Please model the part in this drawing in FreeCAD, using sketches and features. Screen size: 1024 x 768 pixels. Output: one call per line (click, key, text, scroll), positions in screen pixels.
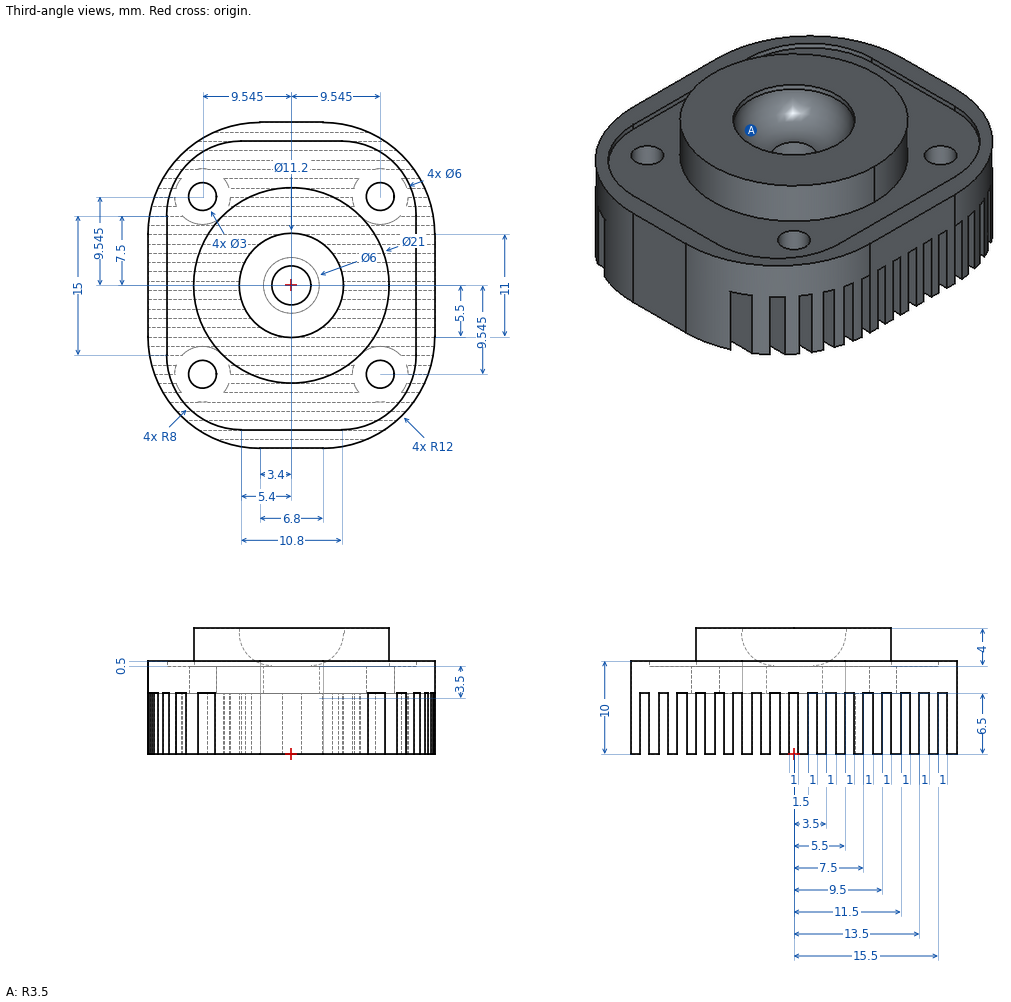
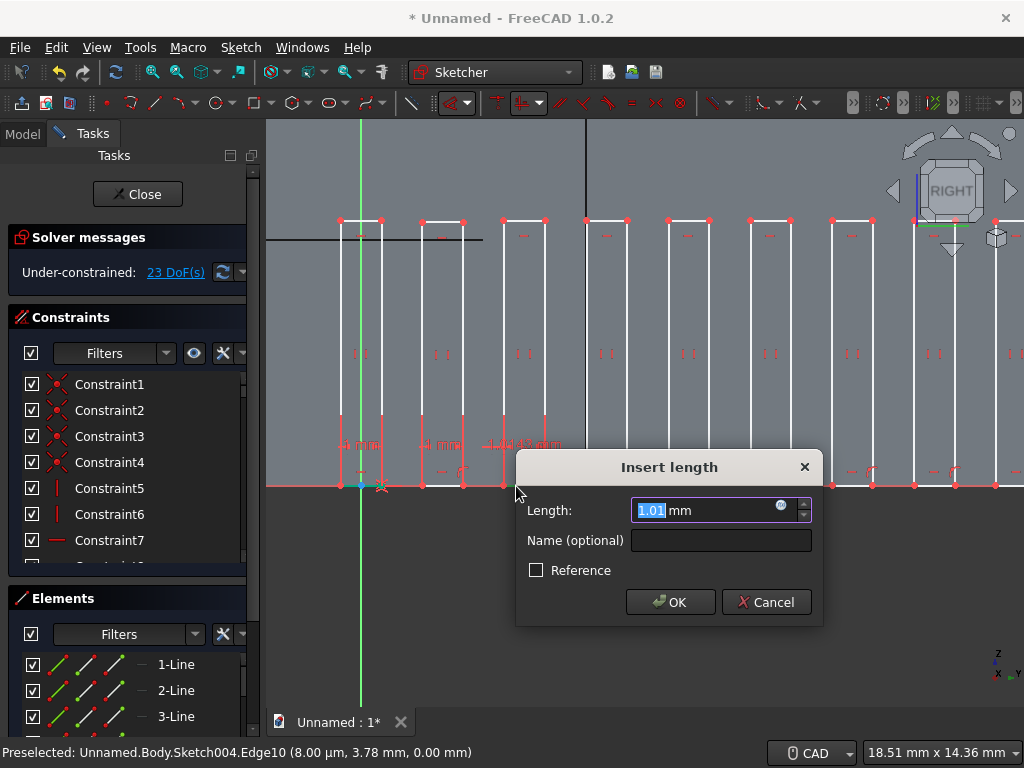
text(1)
key(Return)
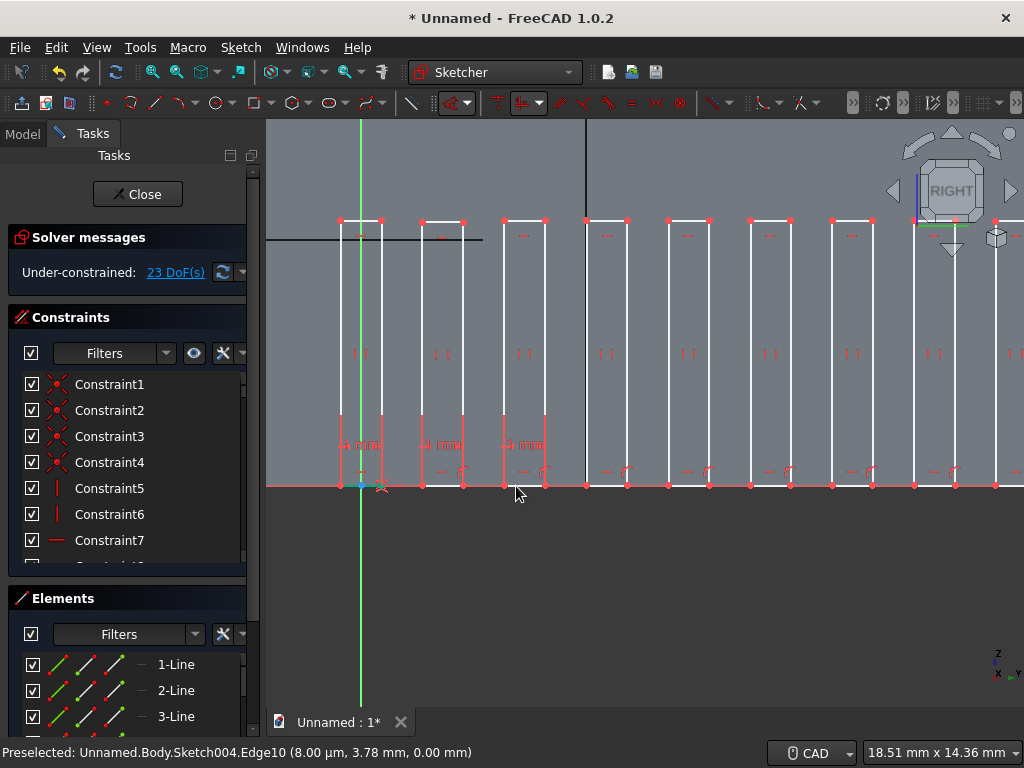
click(599, 486)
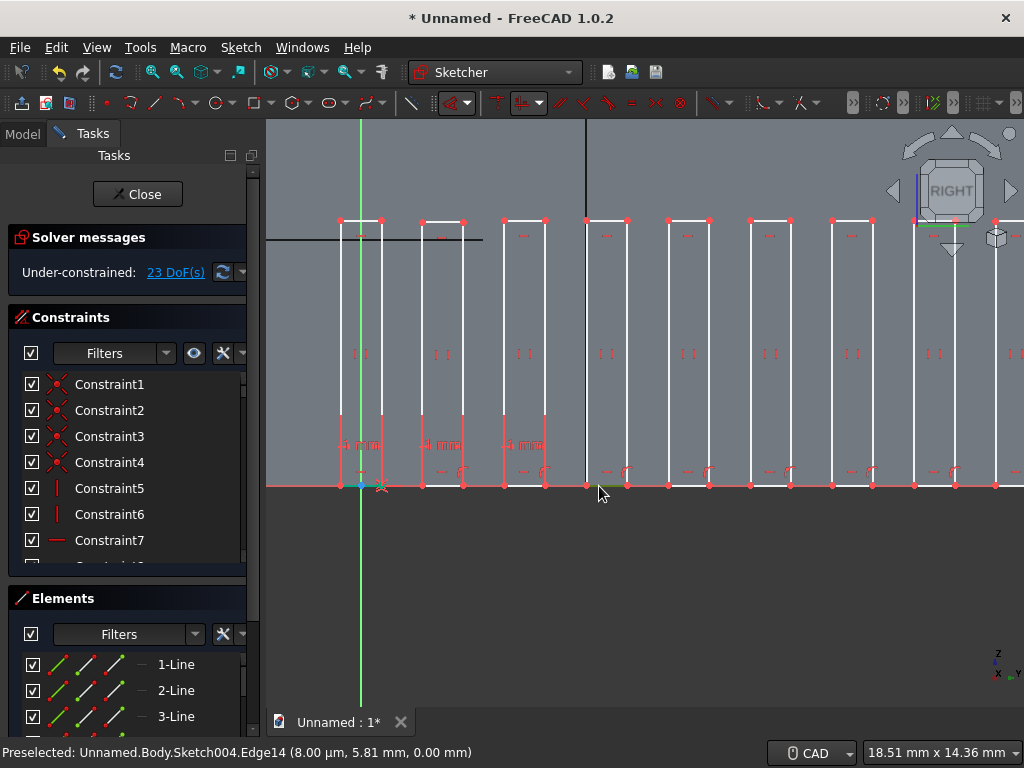
click(470, 104)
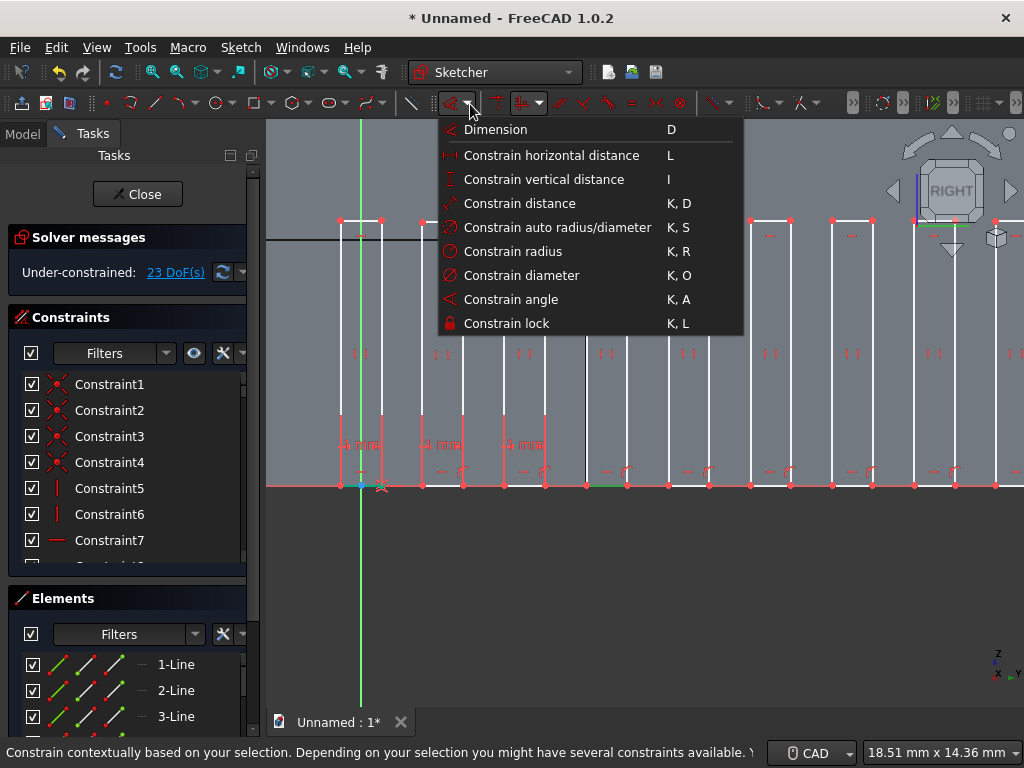
click(591, 155)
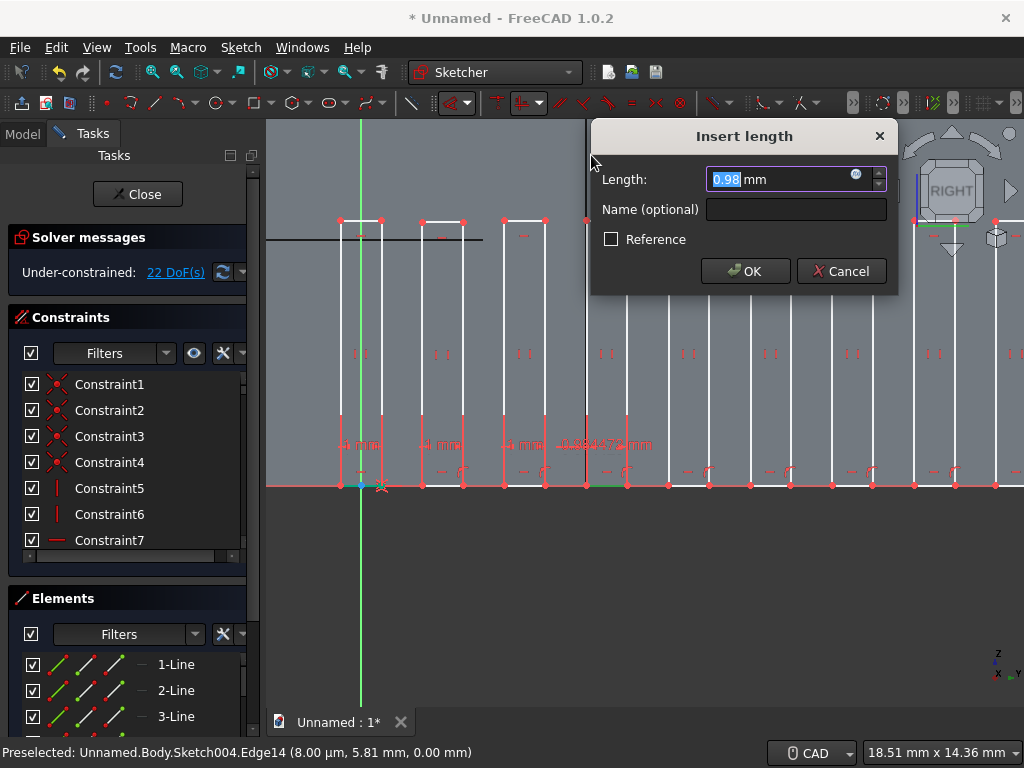
text(1)
key(Return)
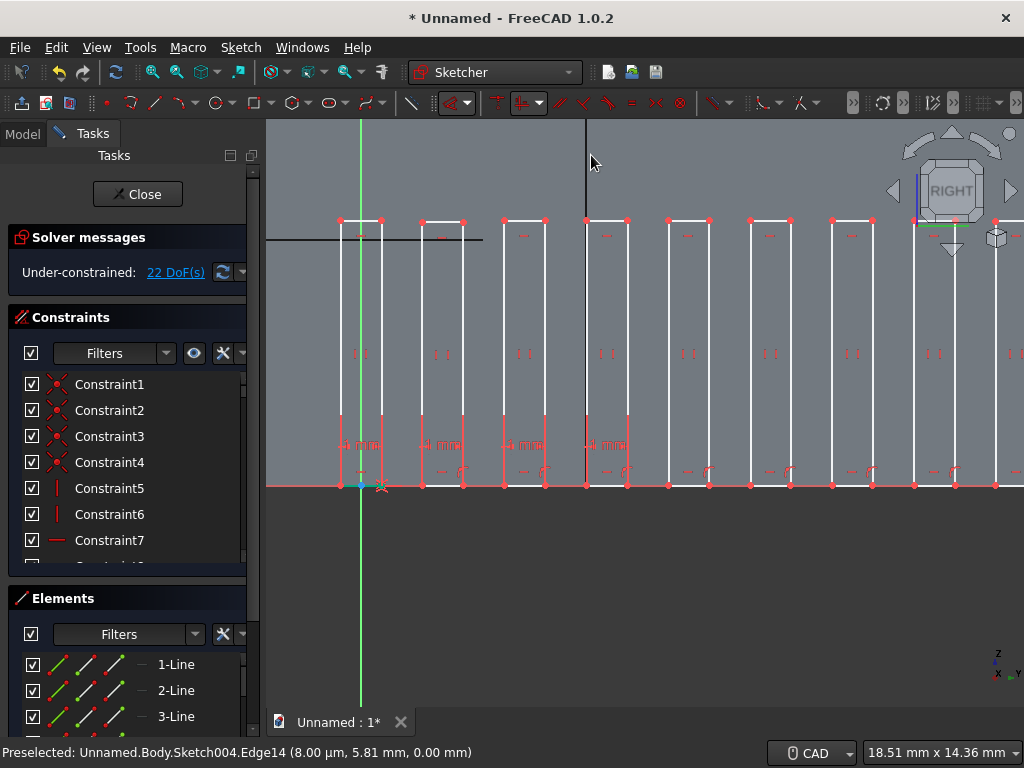
click(681, 486)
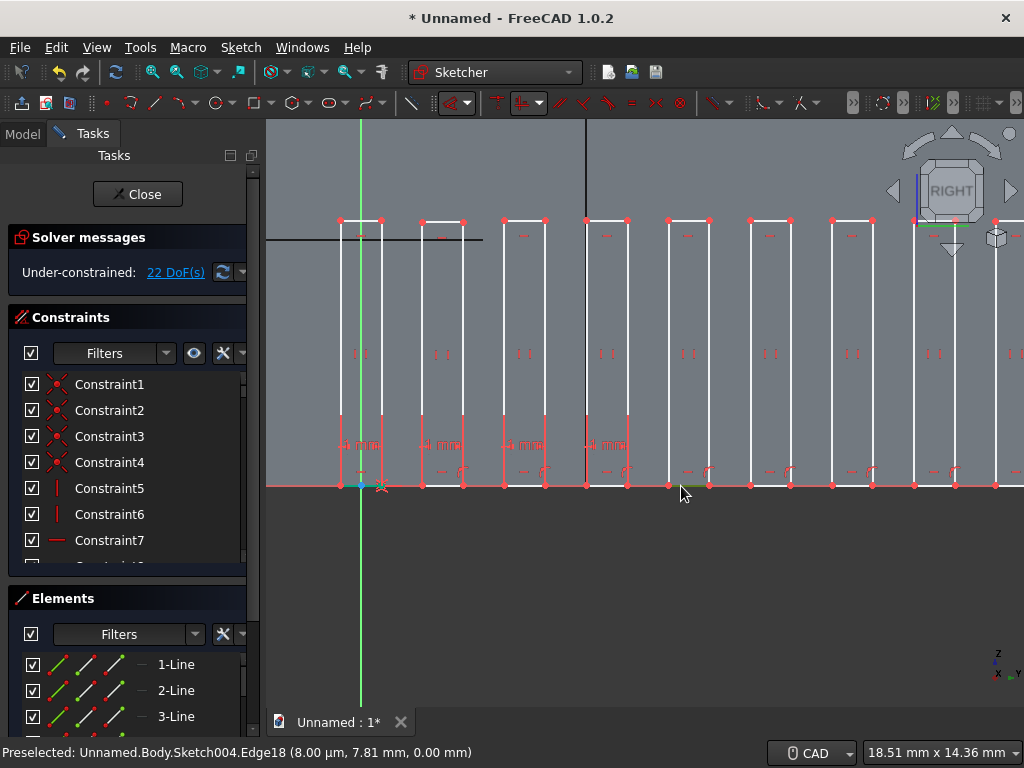
click(470, 104)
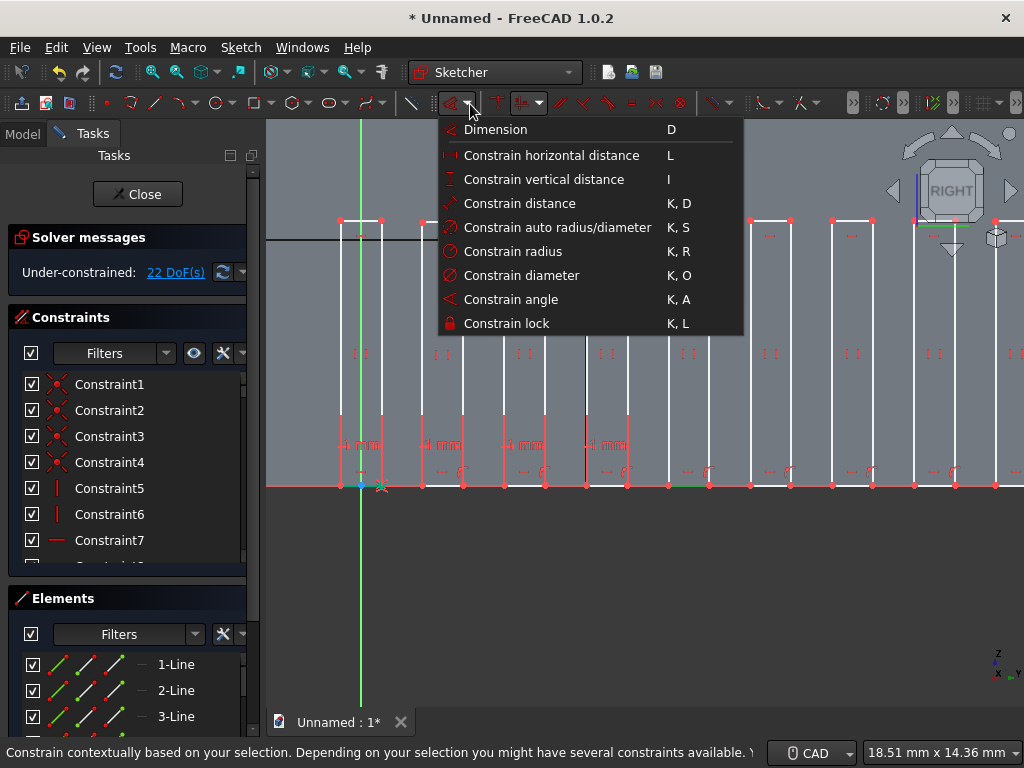
click(591, 155)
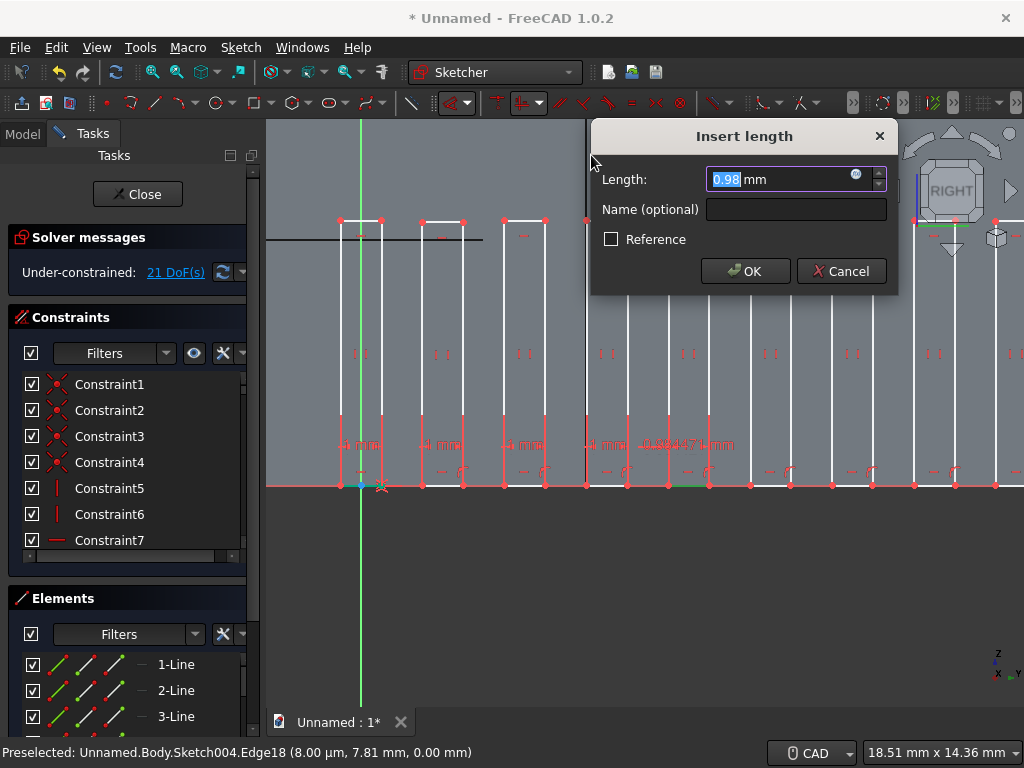
text(1)
key(Return)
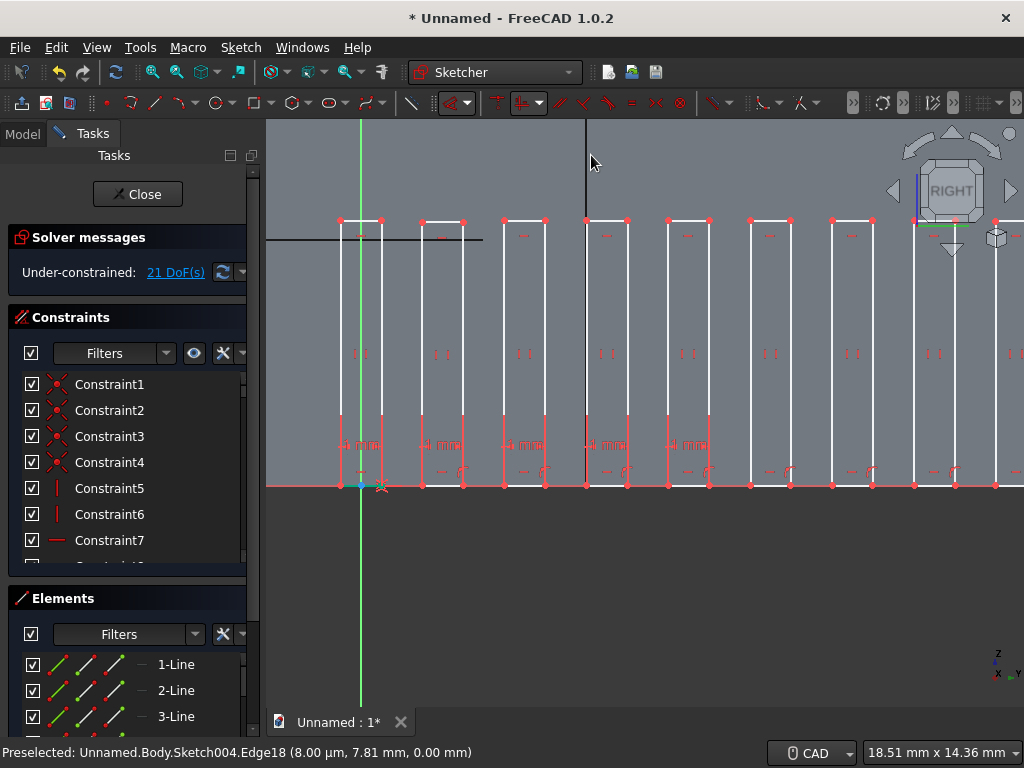
click(763, 486)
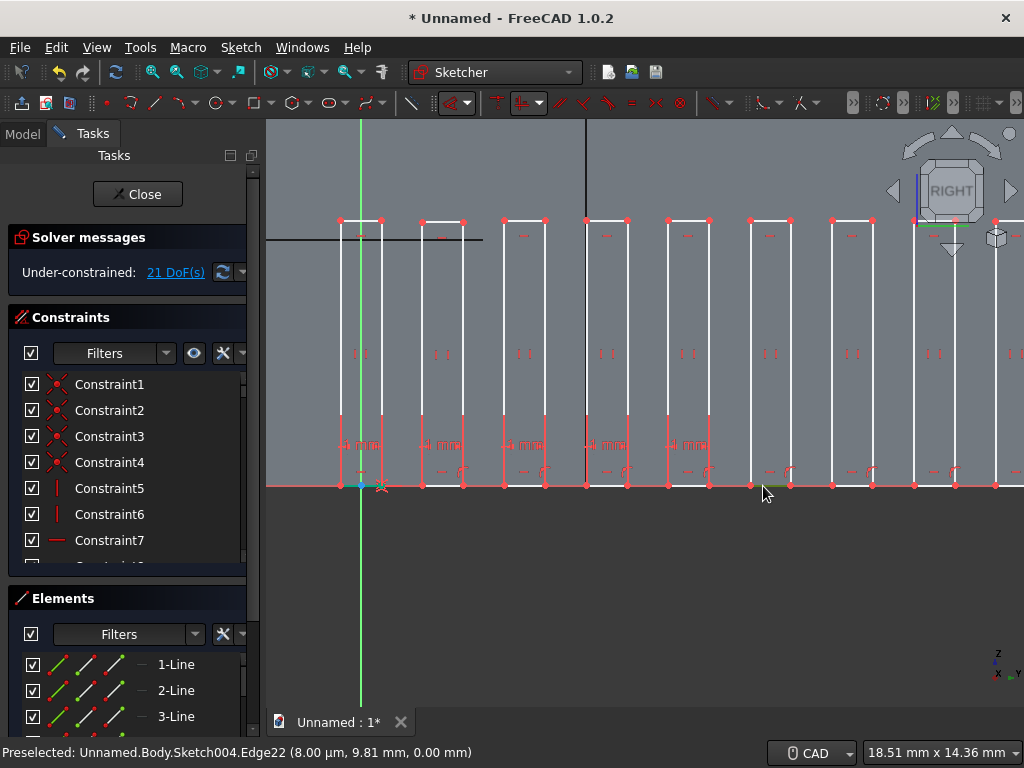
key(l)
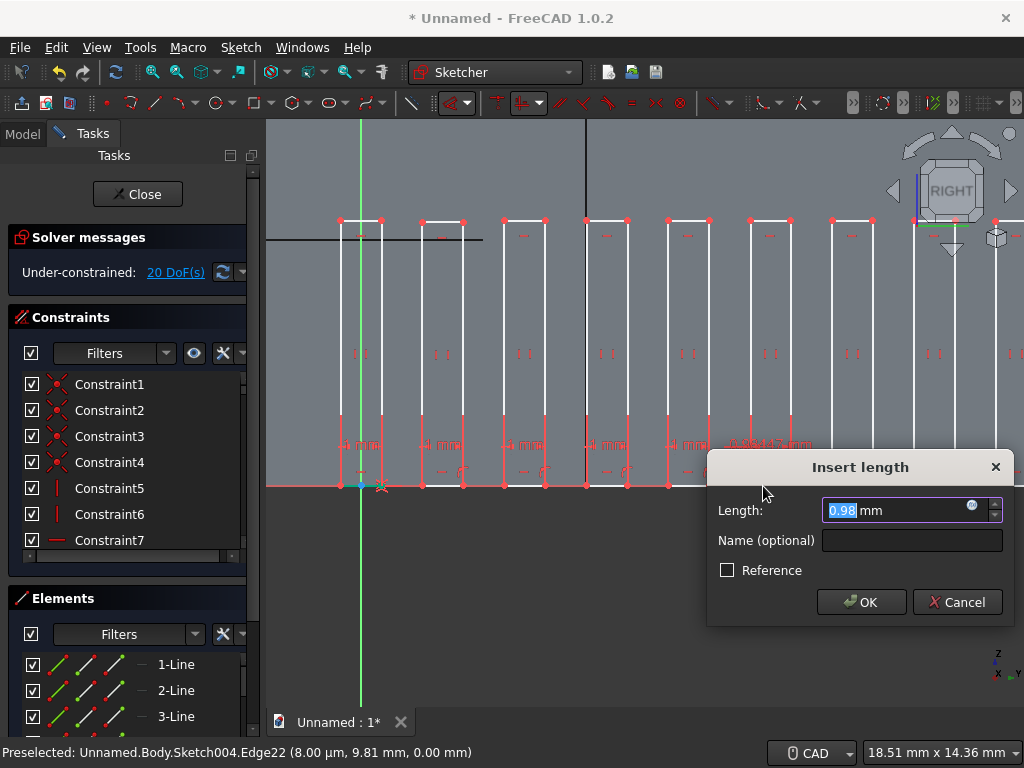
text(1)
key(Return)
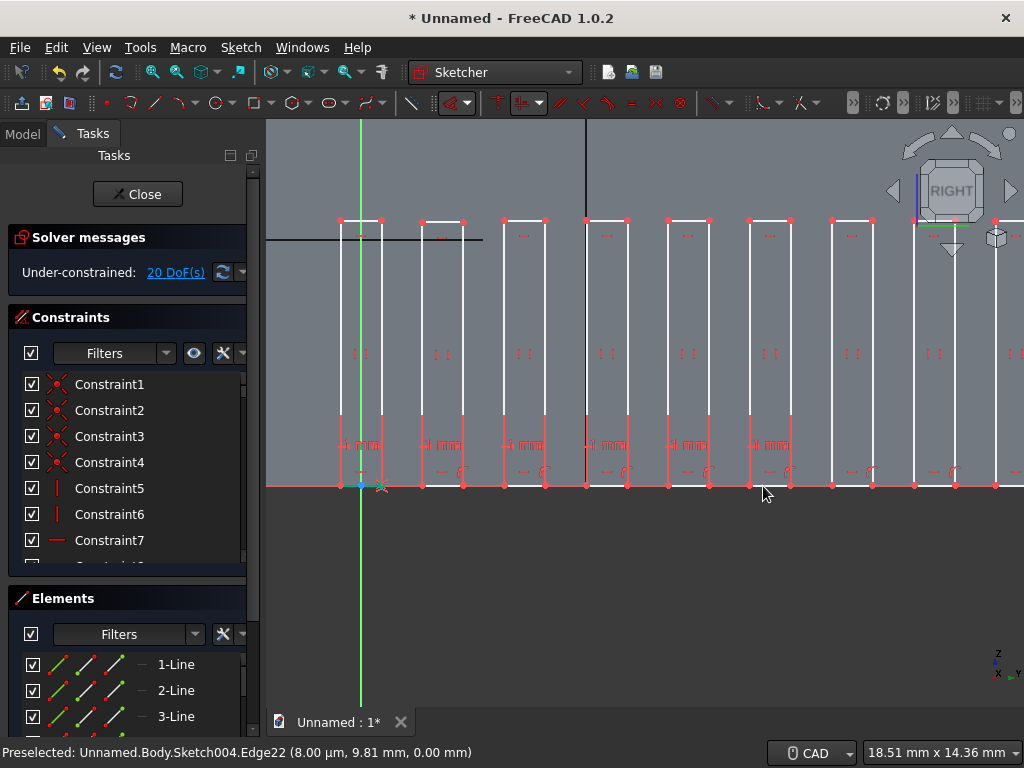
click(845, 486)